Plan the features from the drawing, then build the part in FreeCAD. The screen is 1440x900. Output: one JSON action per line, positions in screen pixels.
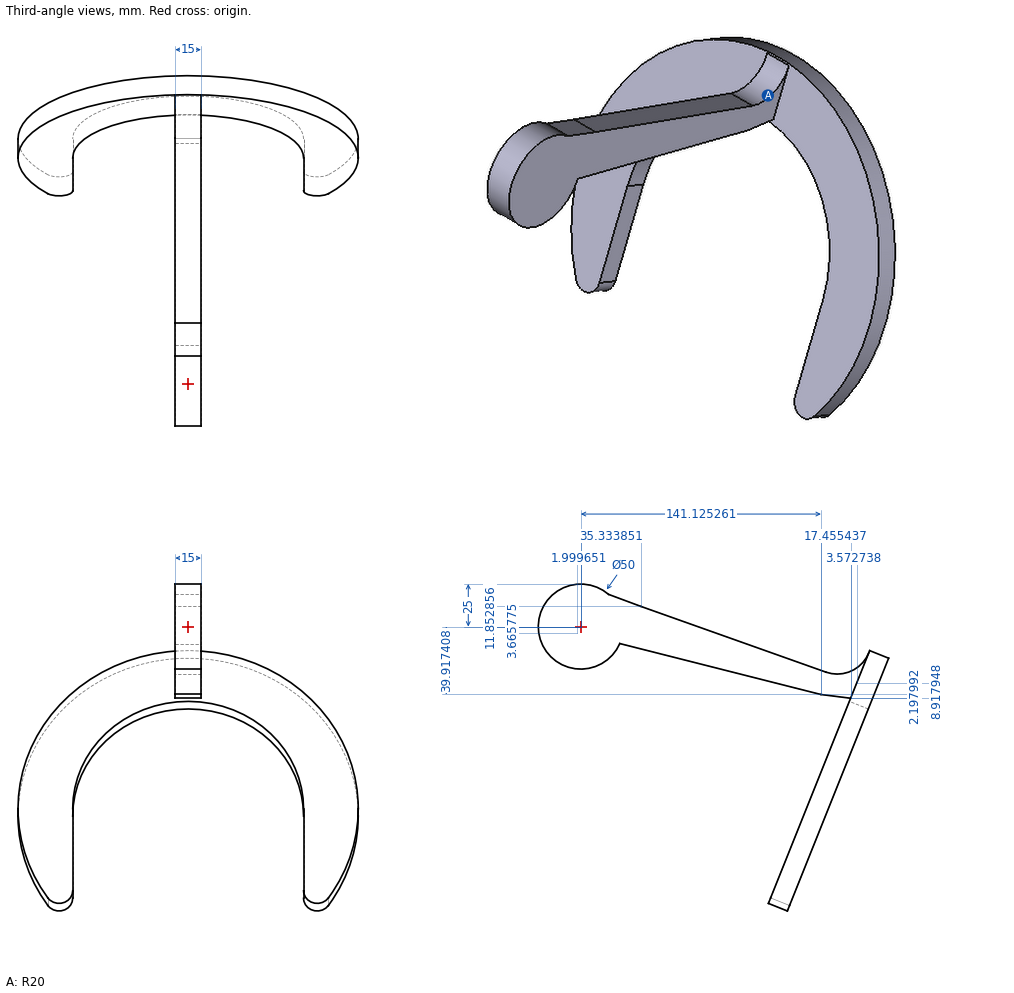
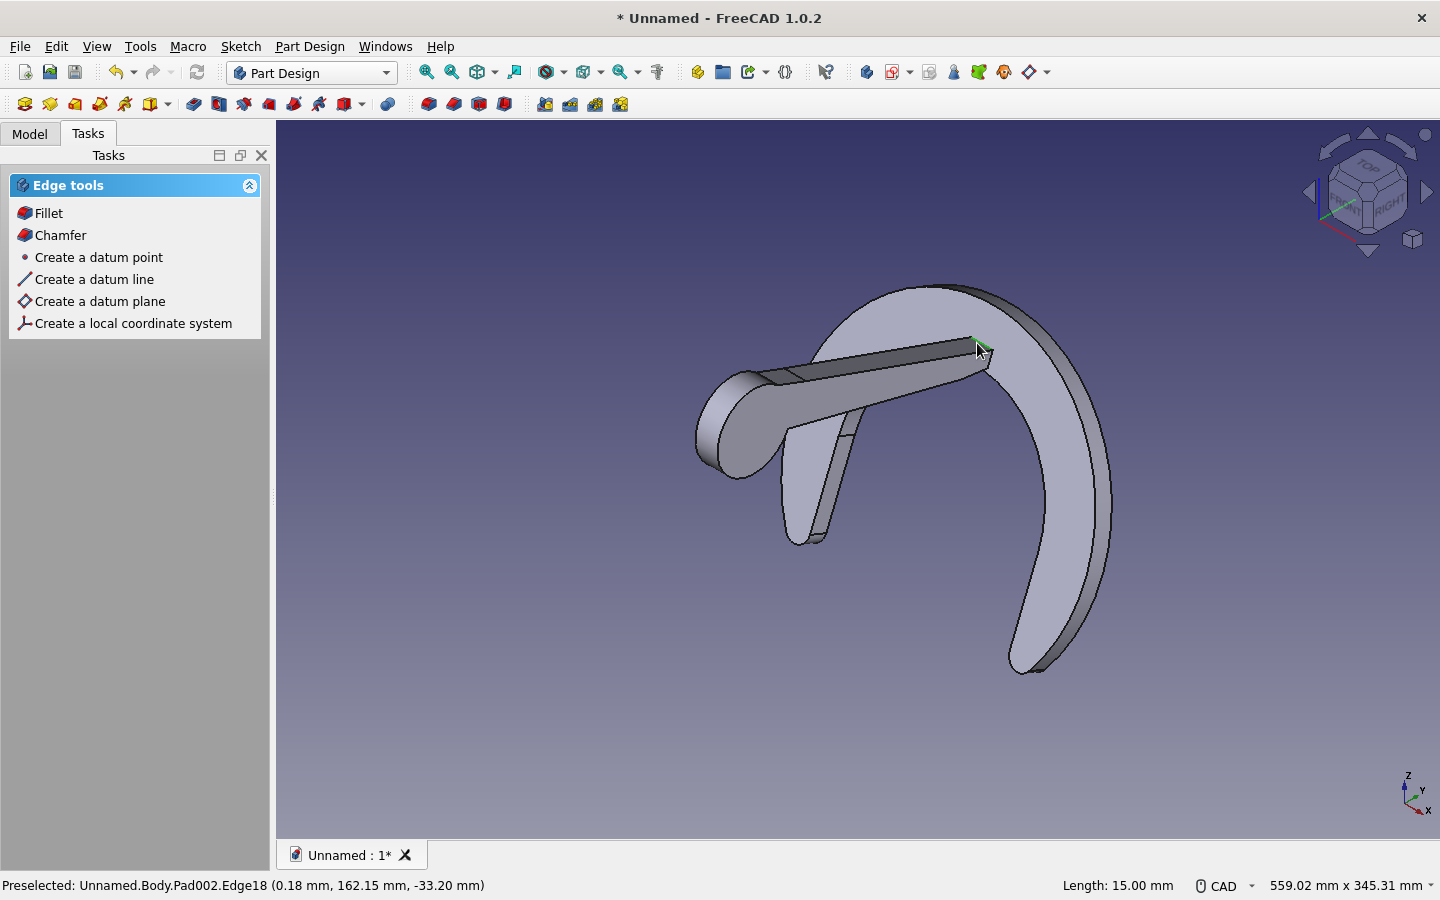
{"action": "left_click", "coordinate": [429, 104]}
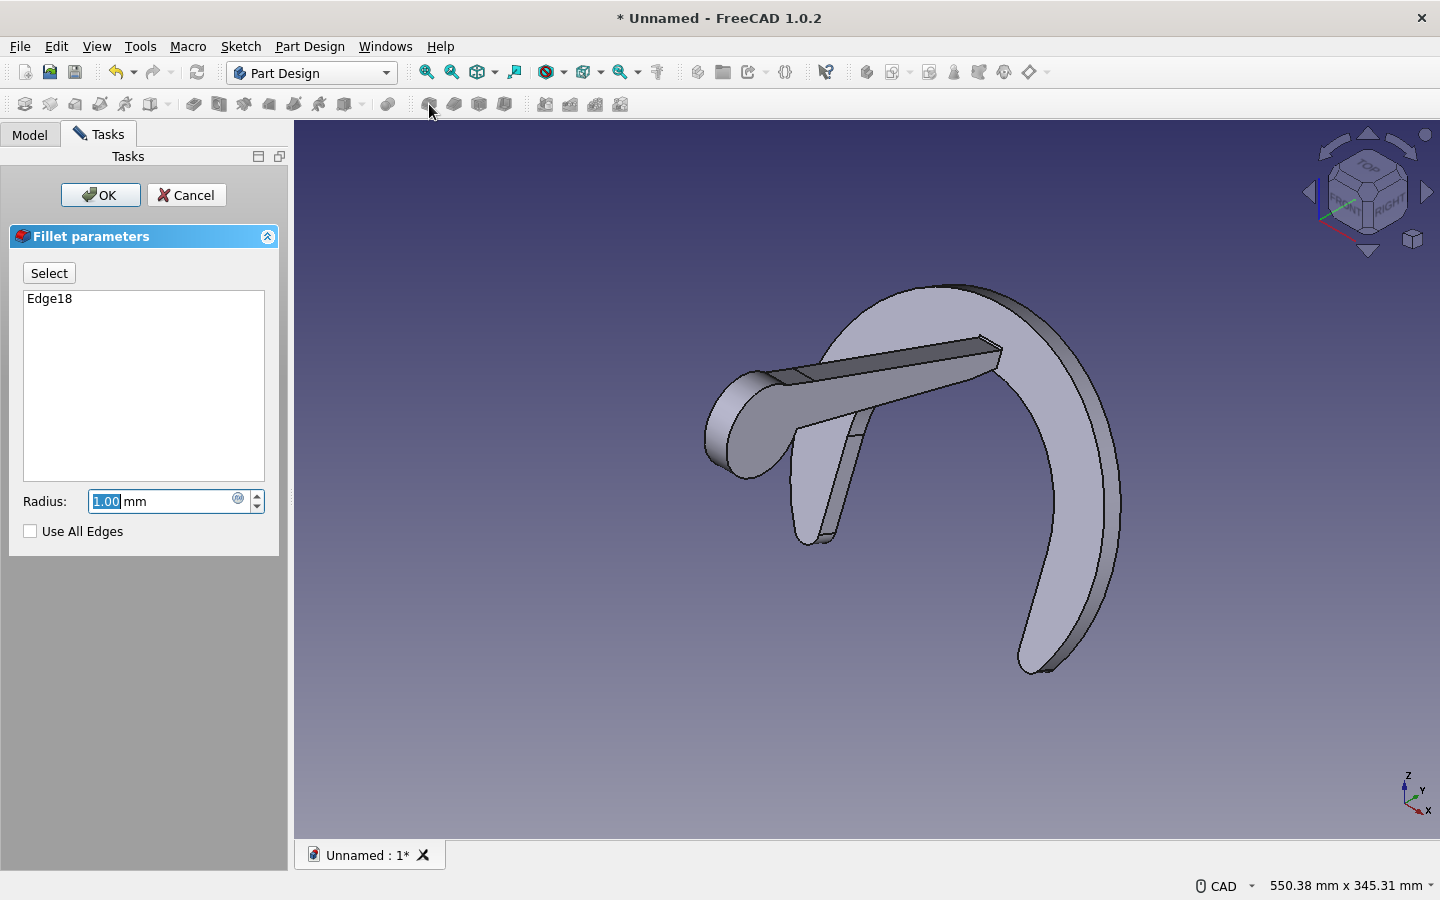
{"action": "type", "text": "20"}
{"action": "key", "text": "Tab"}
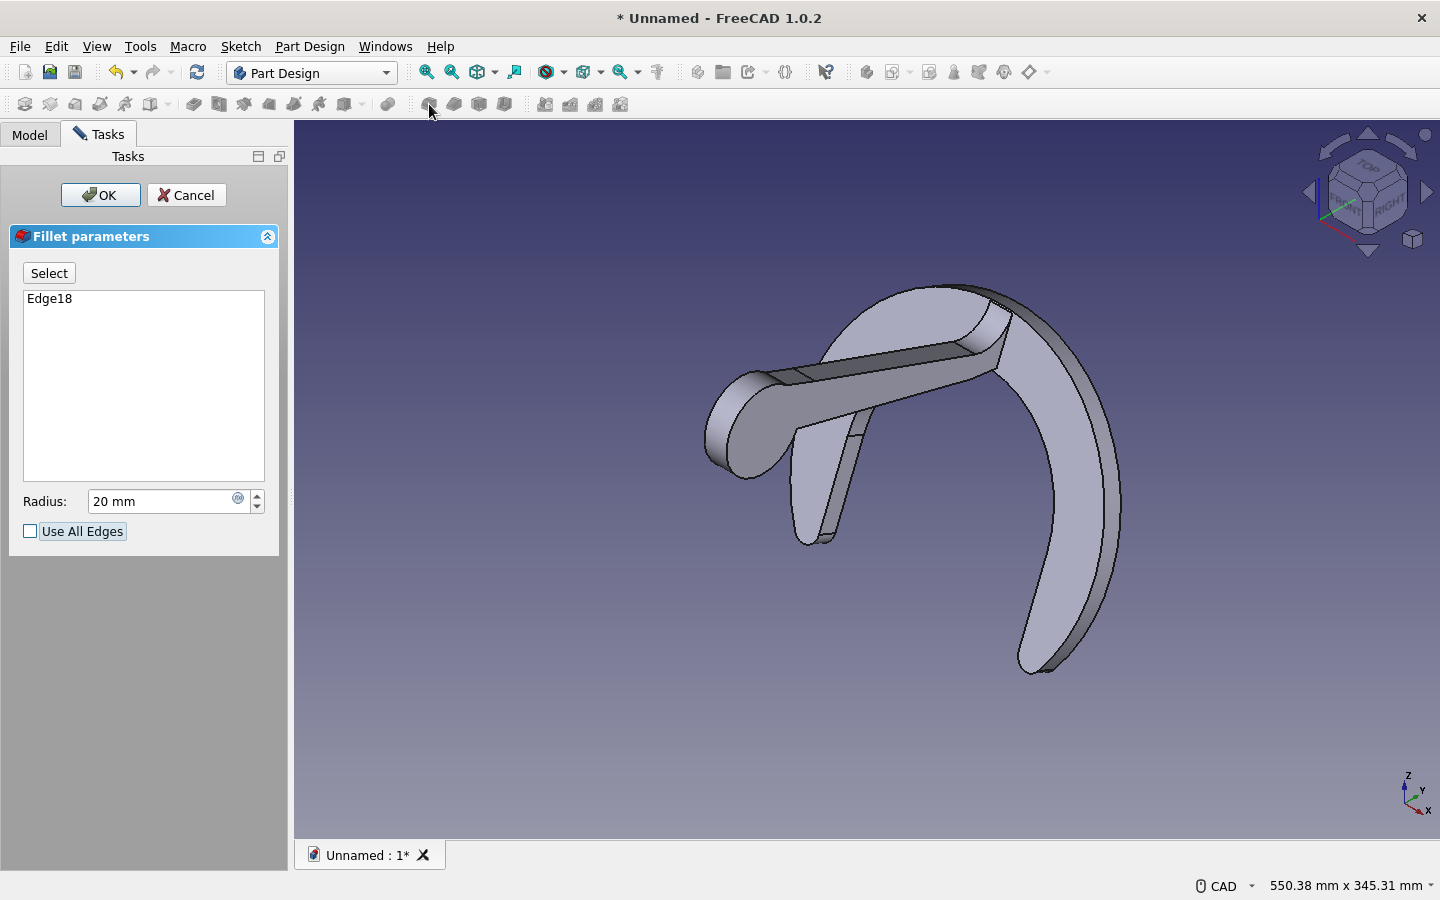
{"action": "left_click", "coordinate": [101, 195]}